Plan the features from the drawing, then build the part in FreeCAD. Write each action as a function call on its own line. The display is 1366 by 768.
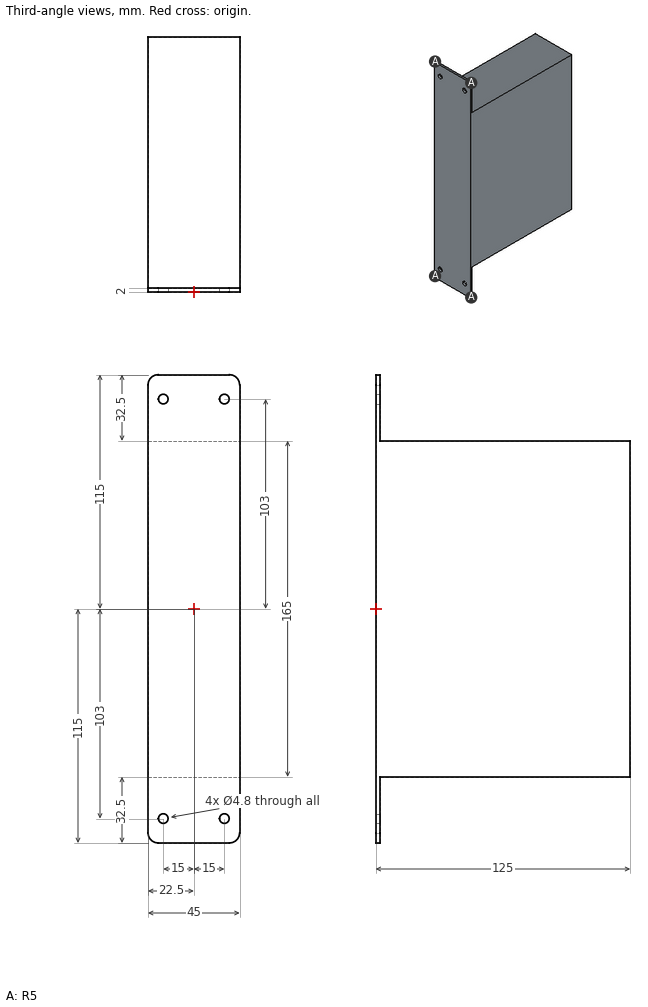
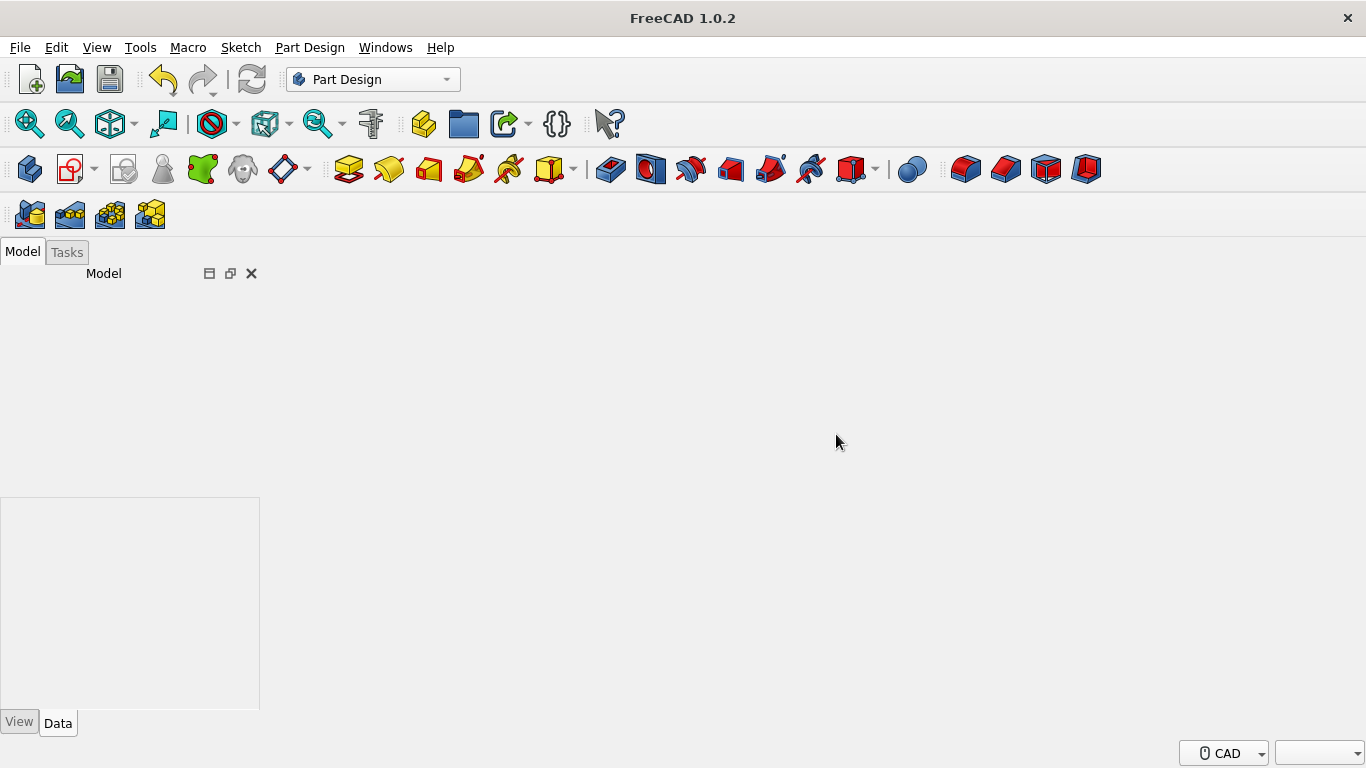
click(30, 80)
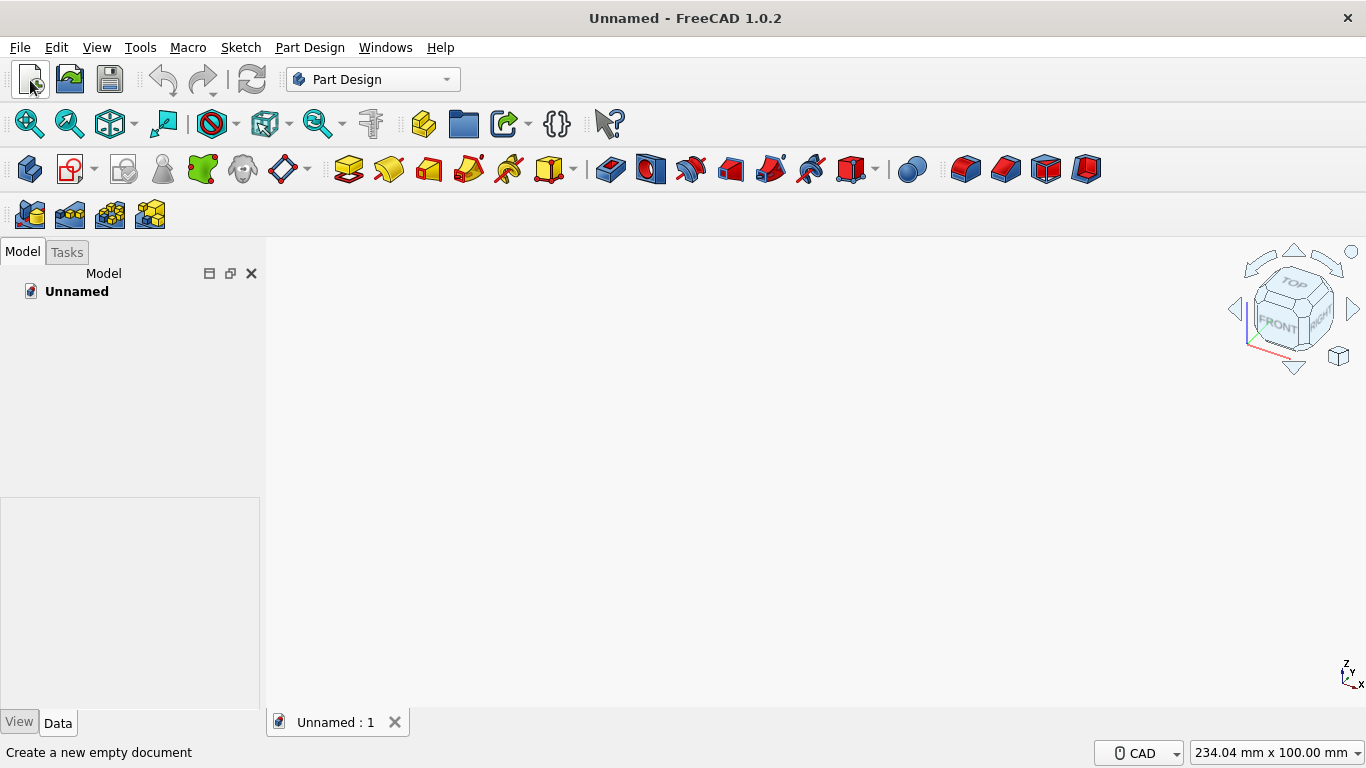
click(70, 170)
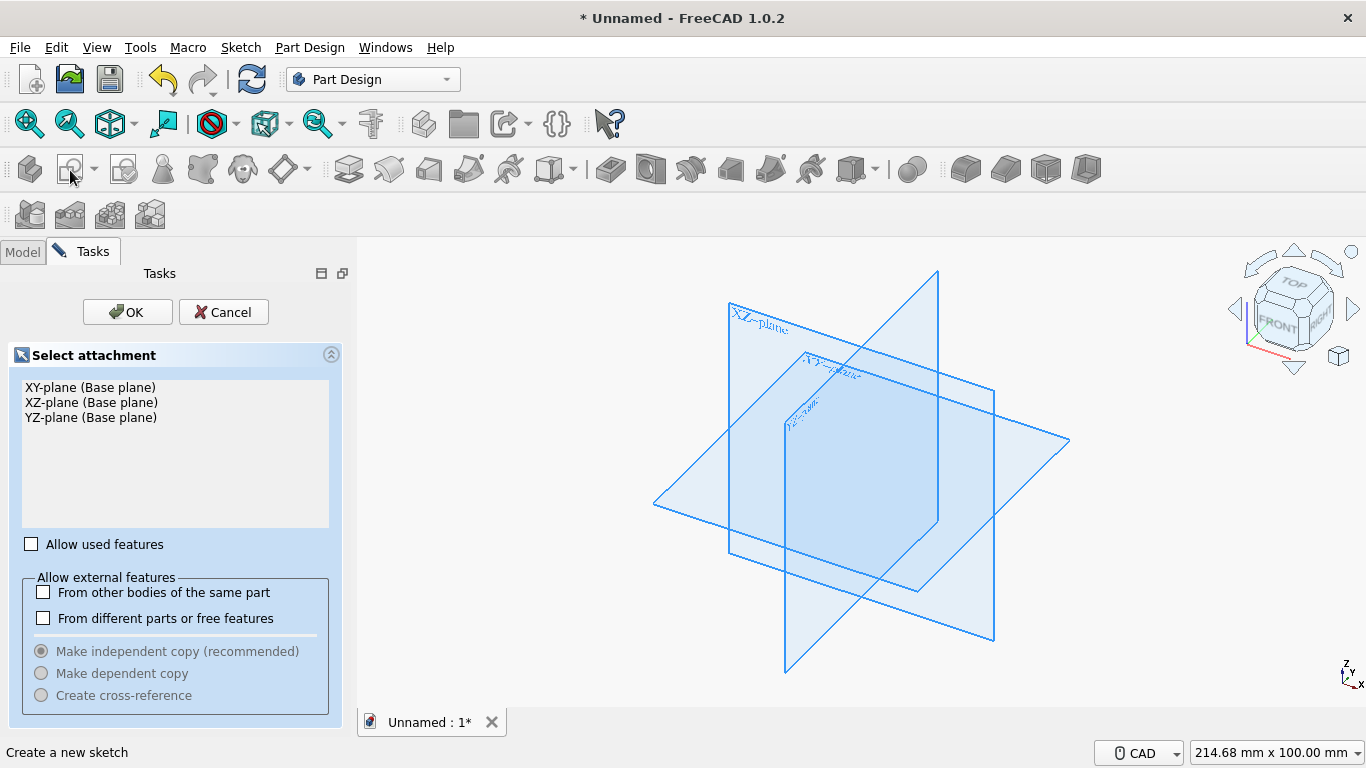
click(82, 402)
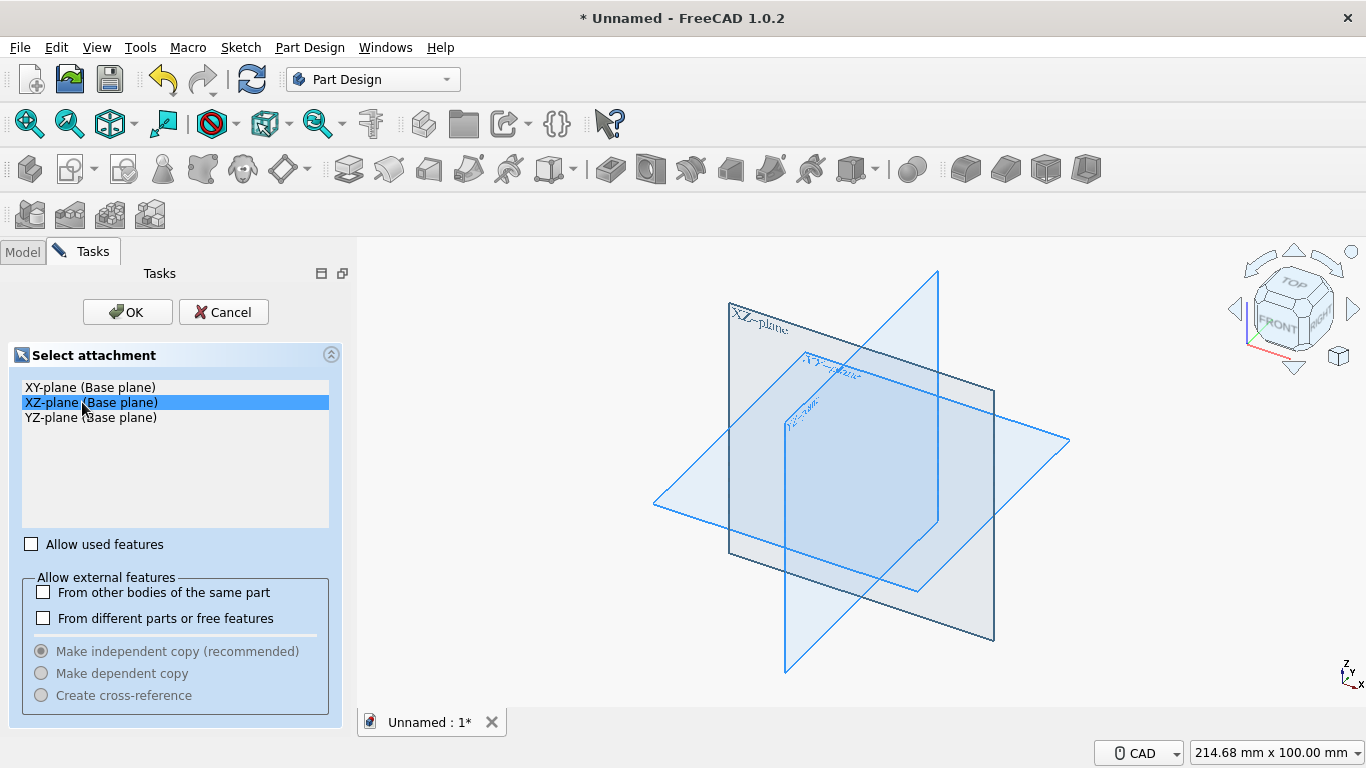
click(128, 312)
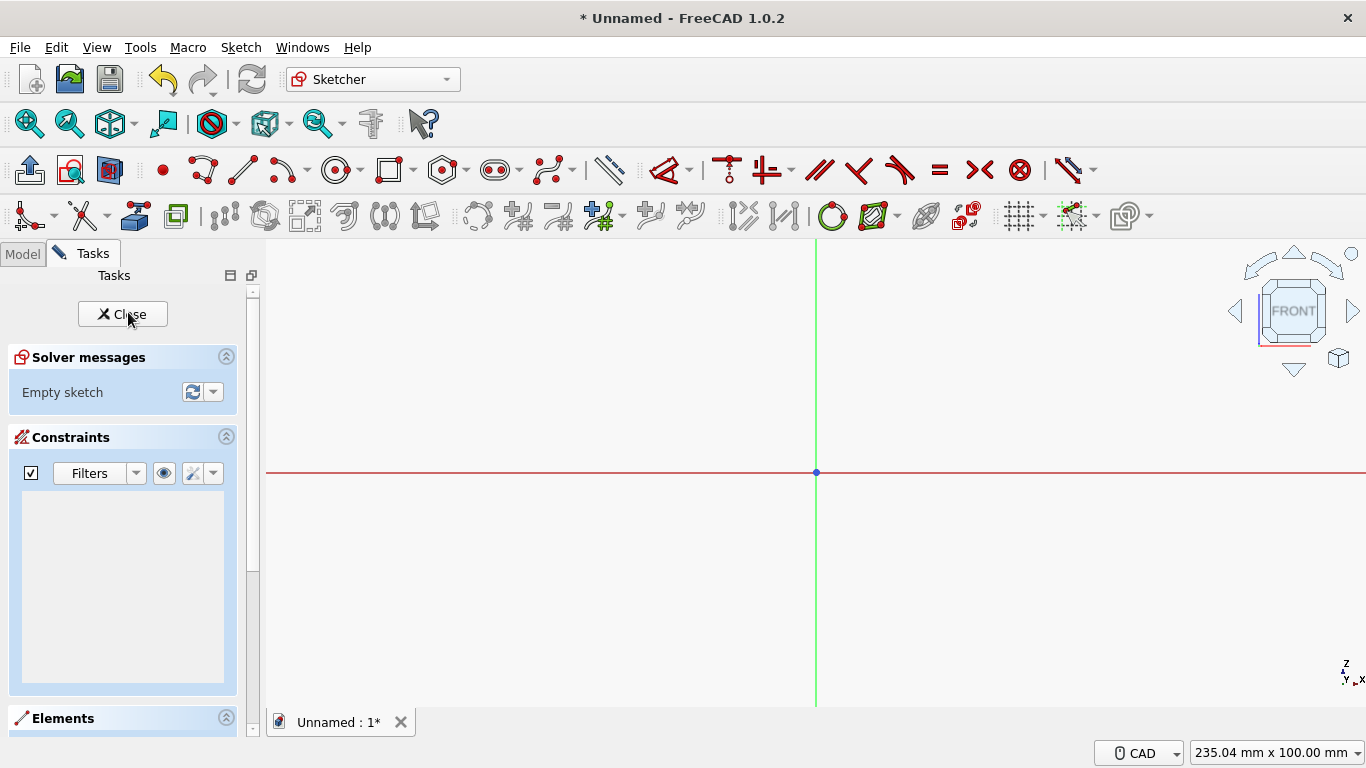
scroll(708, 473, down, 5)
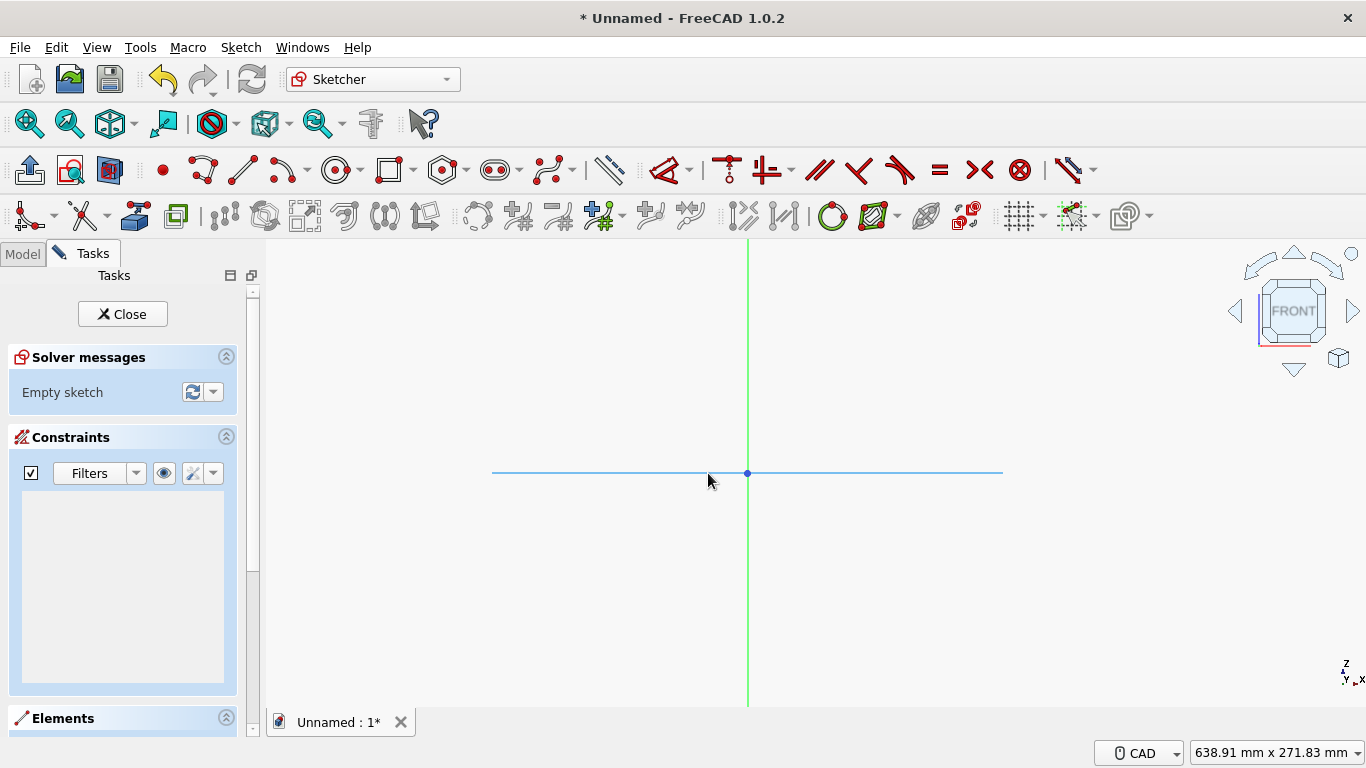
key(g)
key(v)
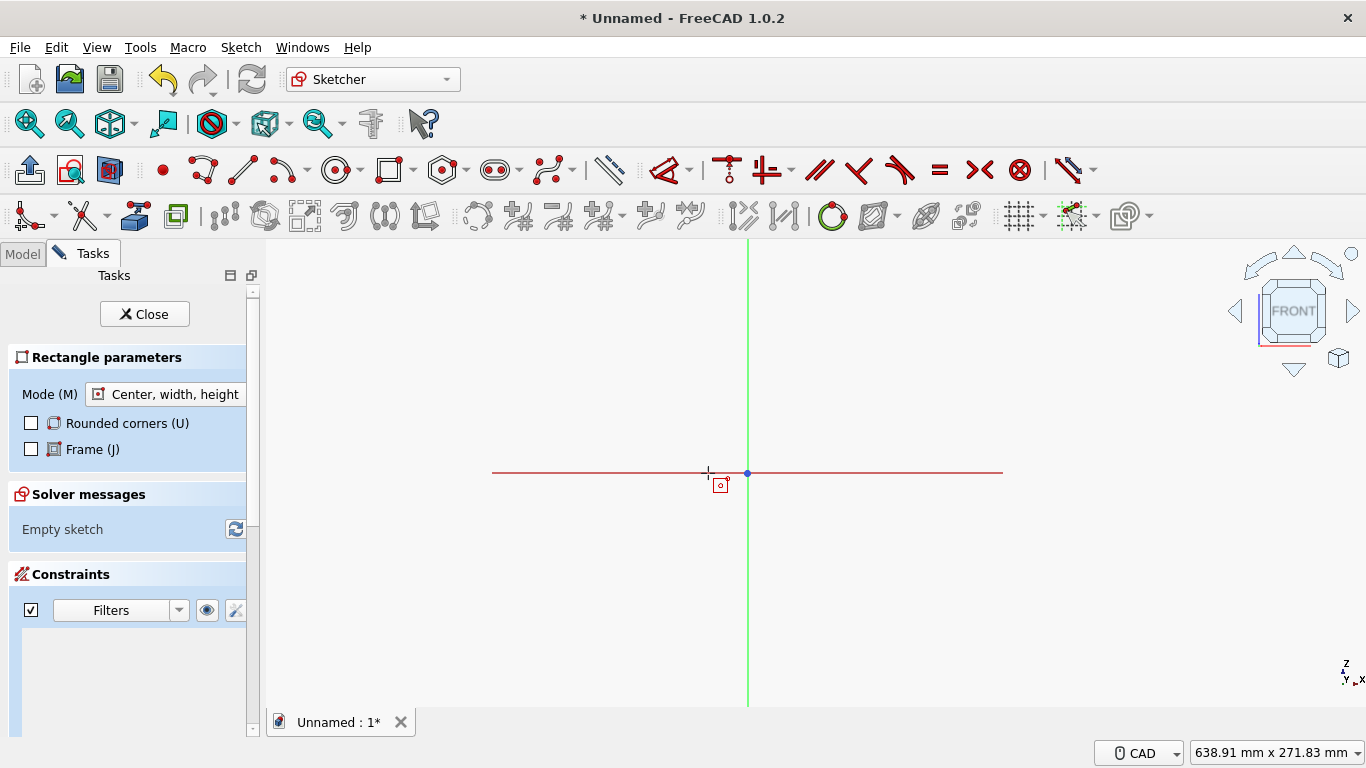
click(748, 473)
click(787, 331)
key(Escape)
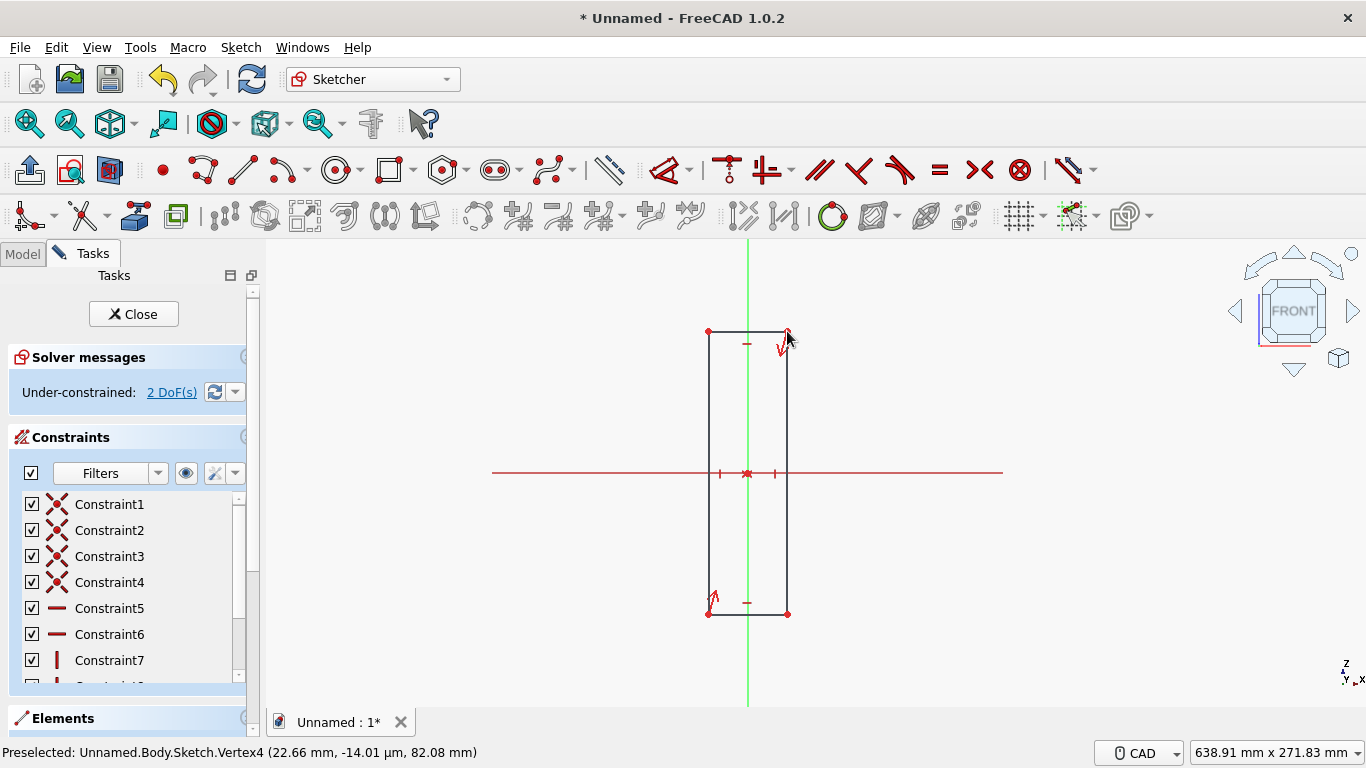
click(732, 615)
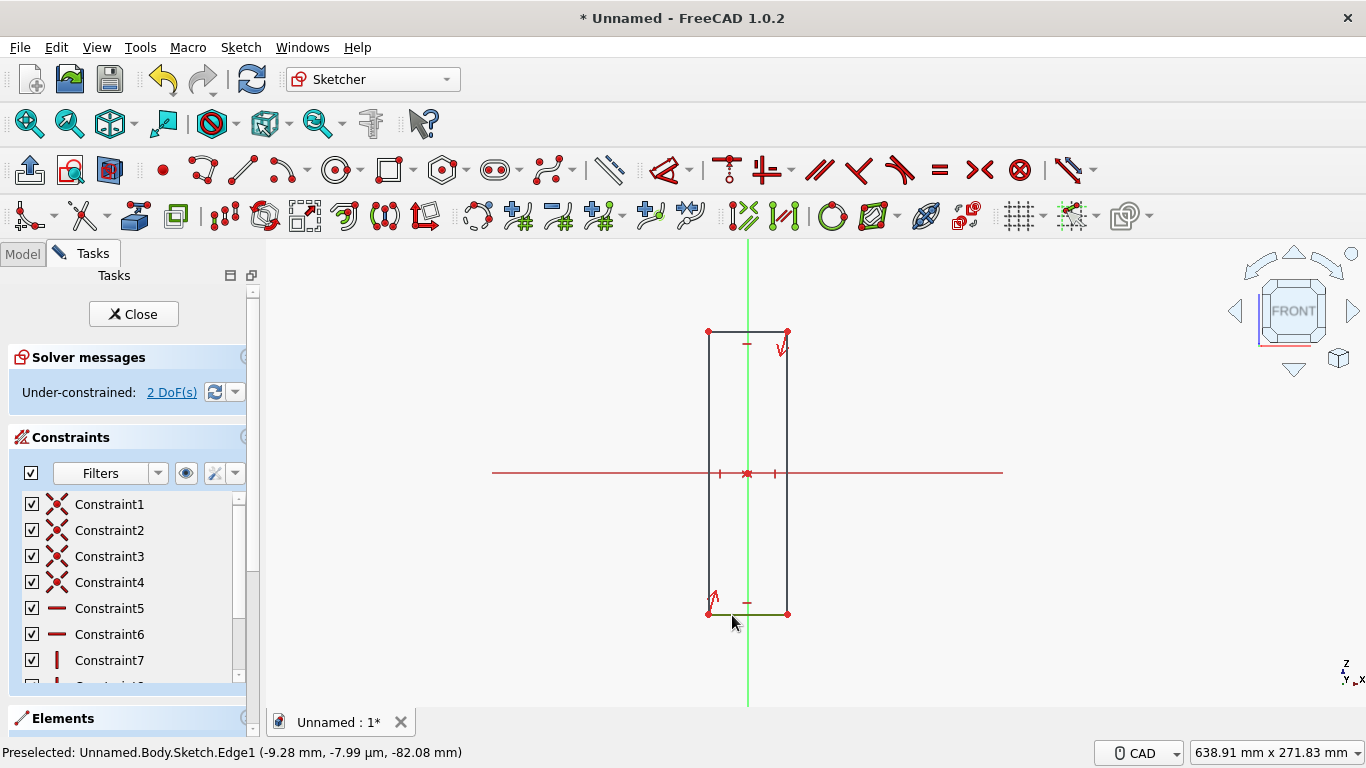
click(692, 170)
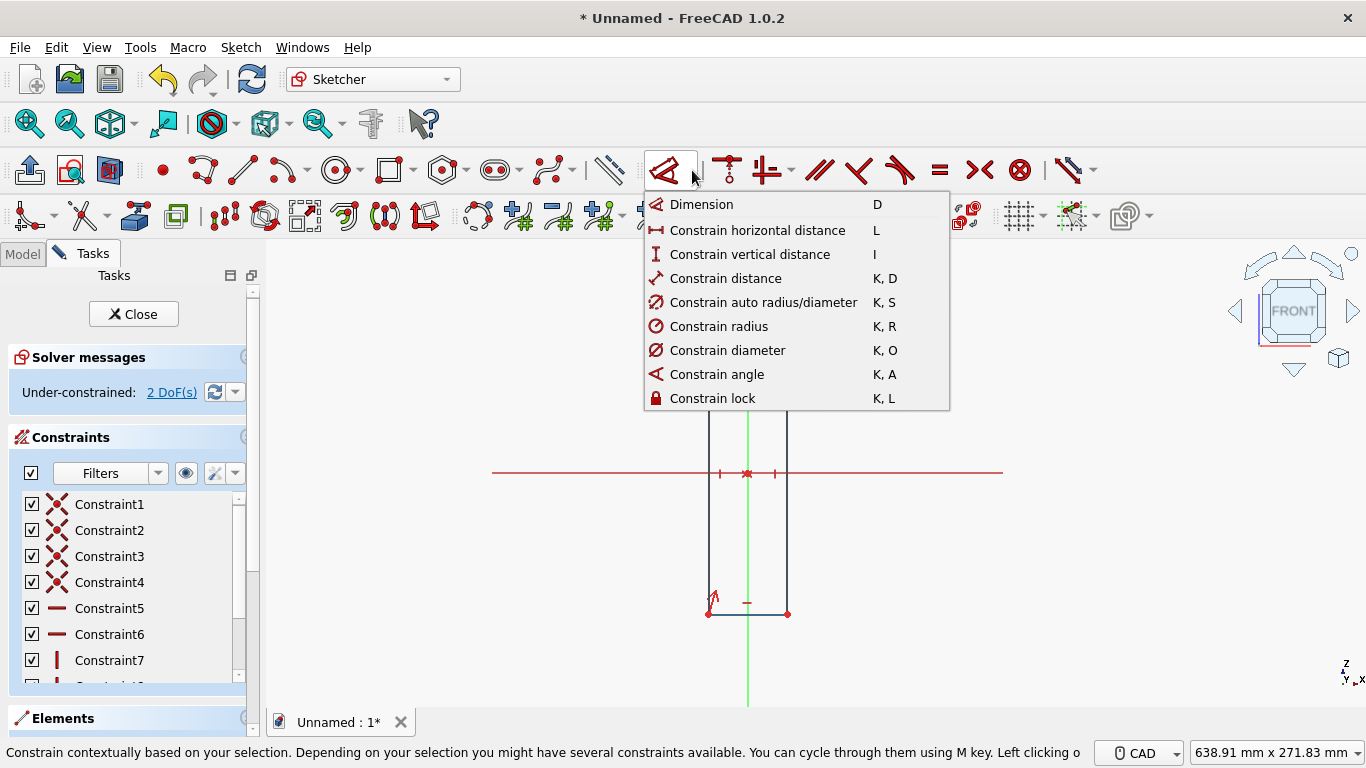
click(797, 230)